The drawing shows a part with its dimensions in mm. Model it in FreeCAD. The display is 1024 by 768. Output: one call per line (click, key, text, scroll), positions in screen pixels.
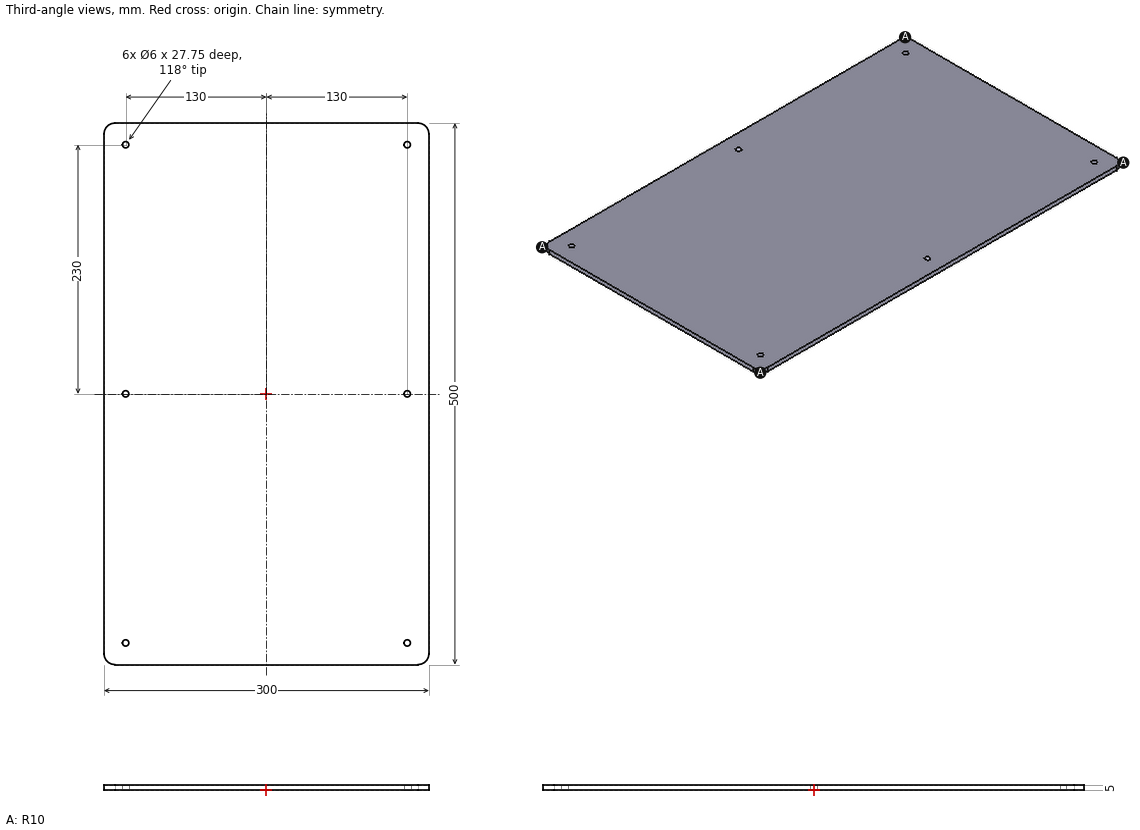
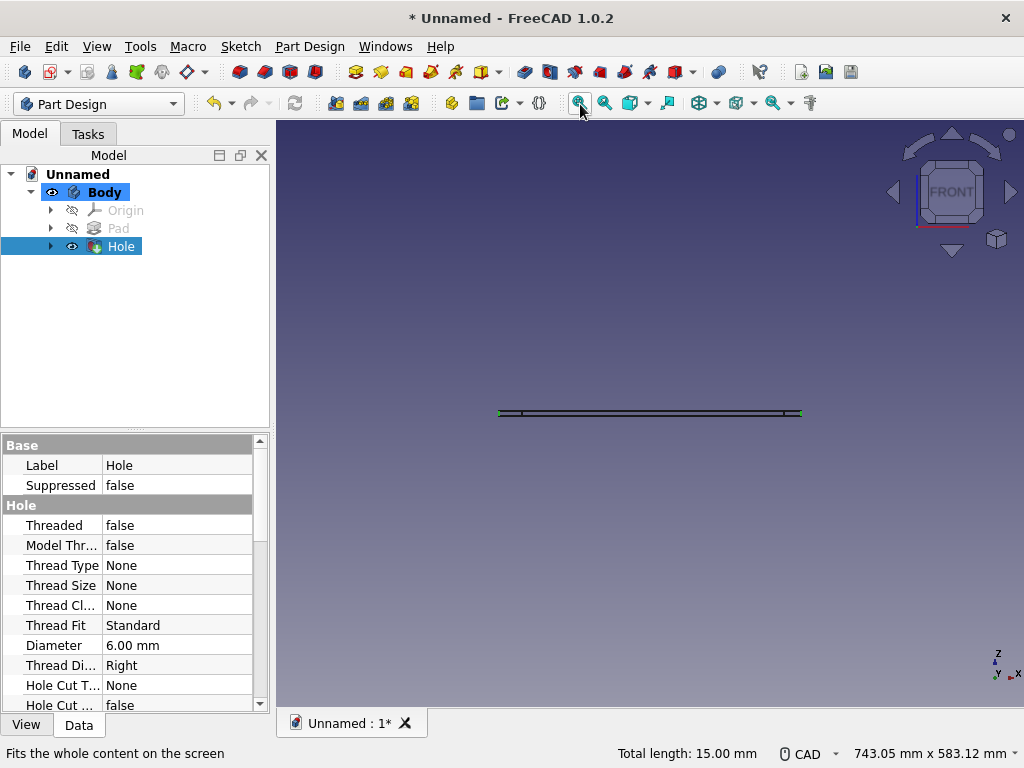
click(580, 104)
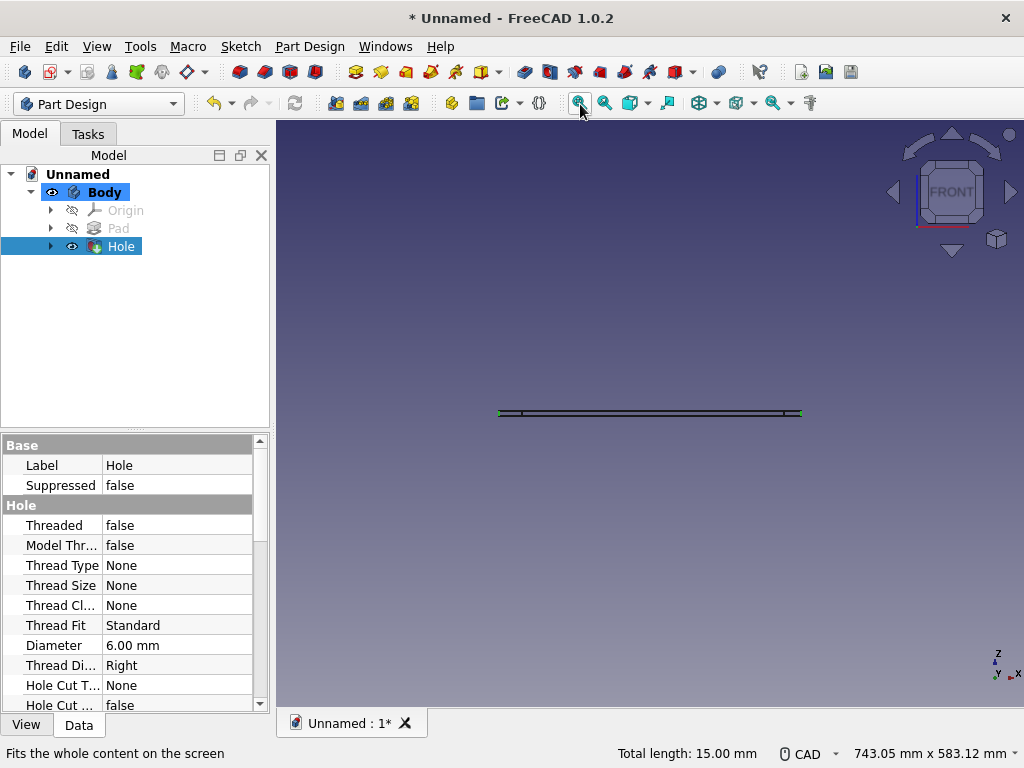
scroll(801, 413, up, 11)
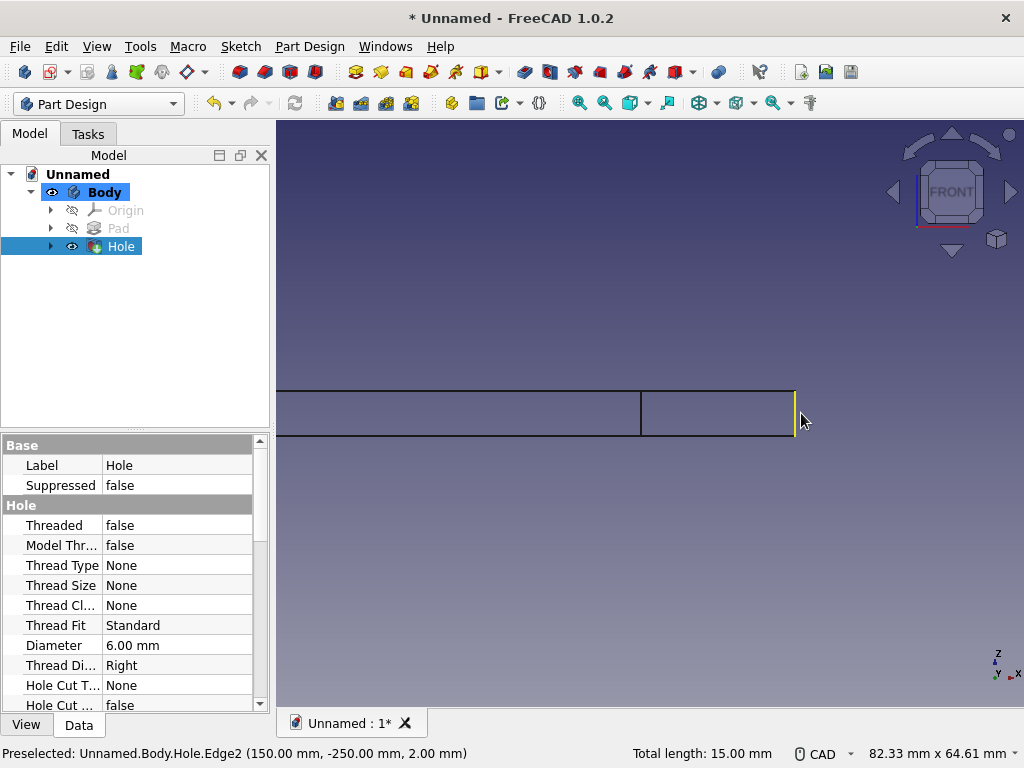
click(580, 104)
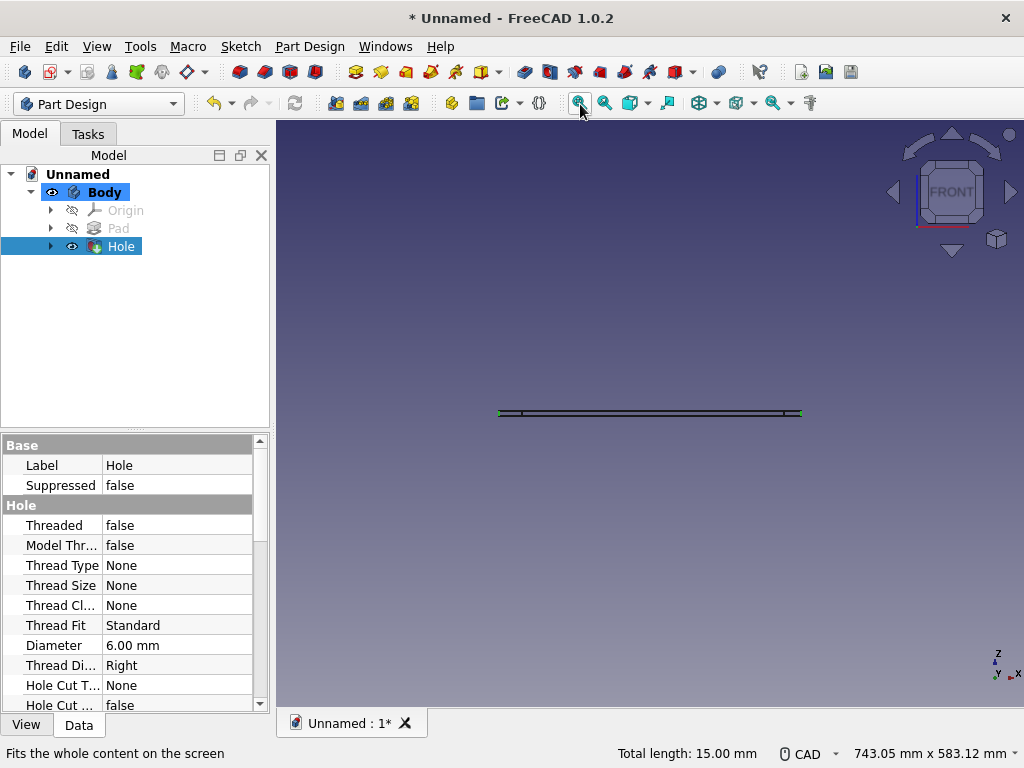
key(3)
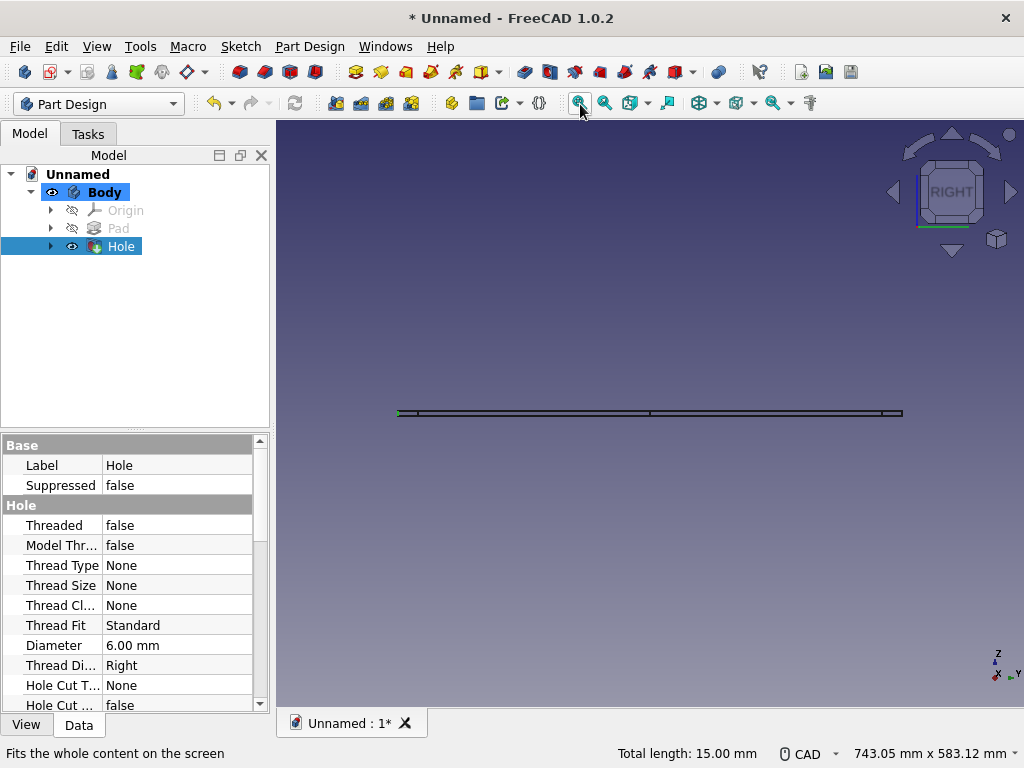
key(5)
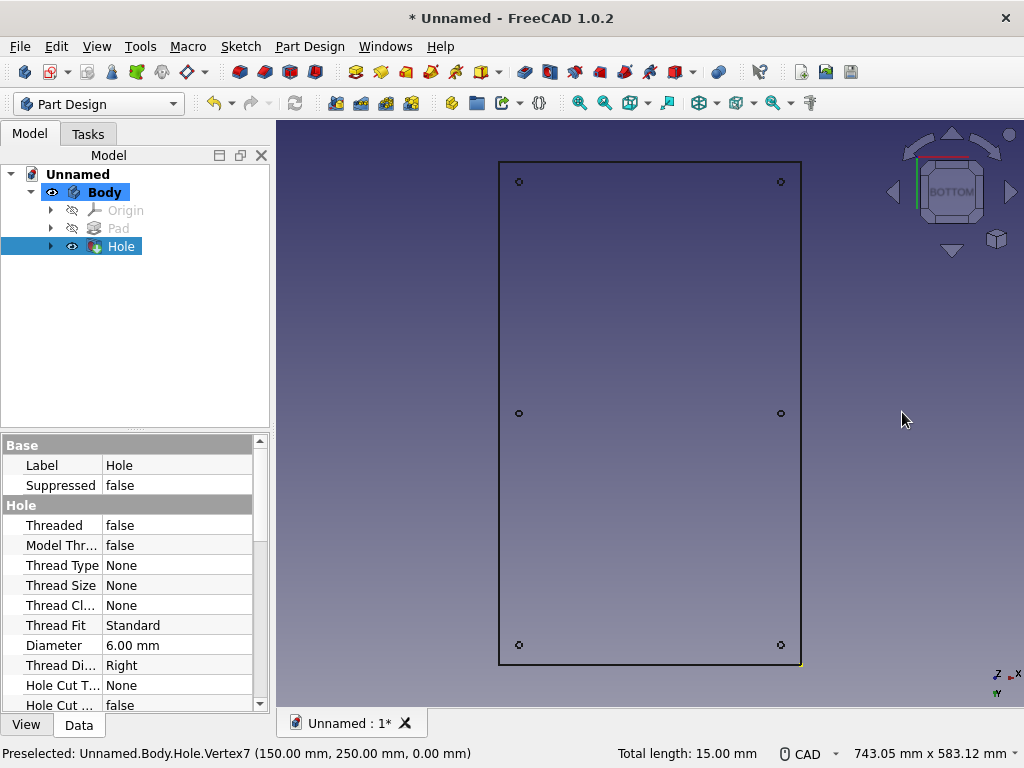
scroll(801, 664, up, 11)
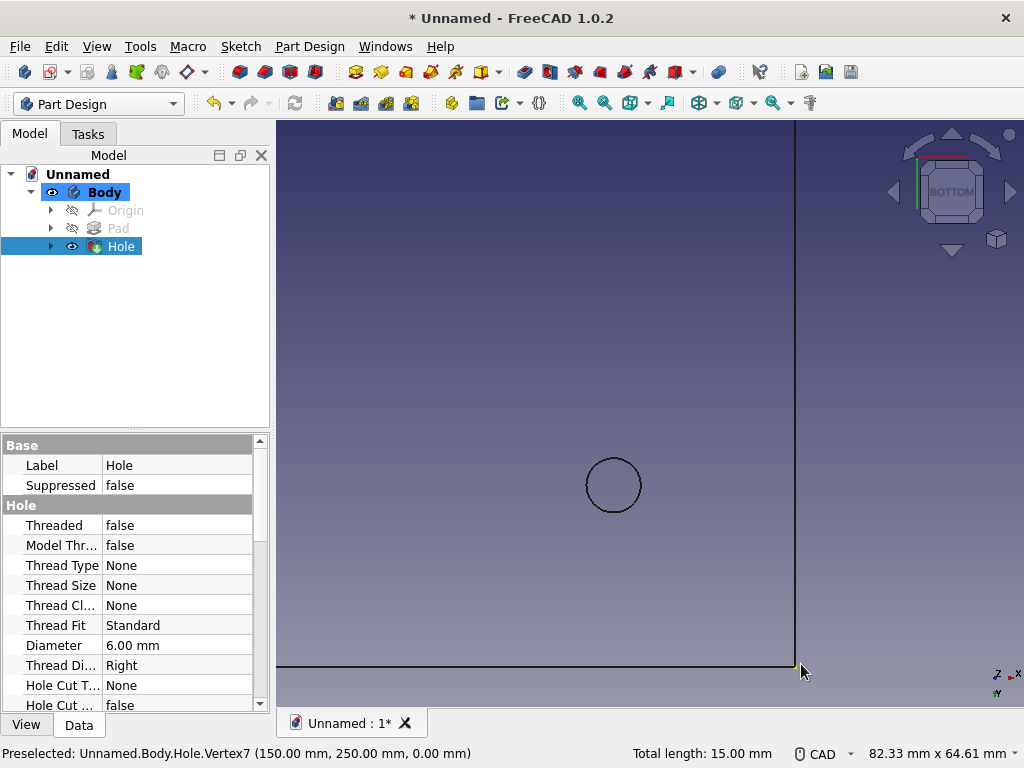
click(580, 104)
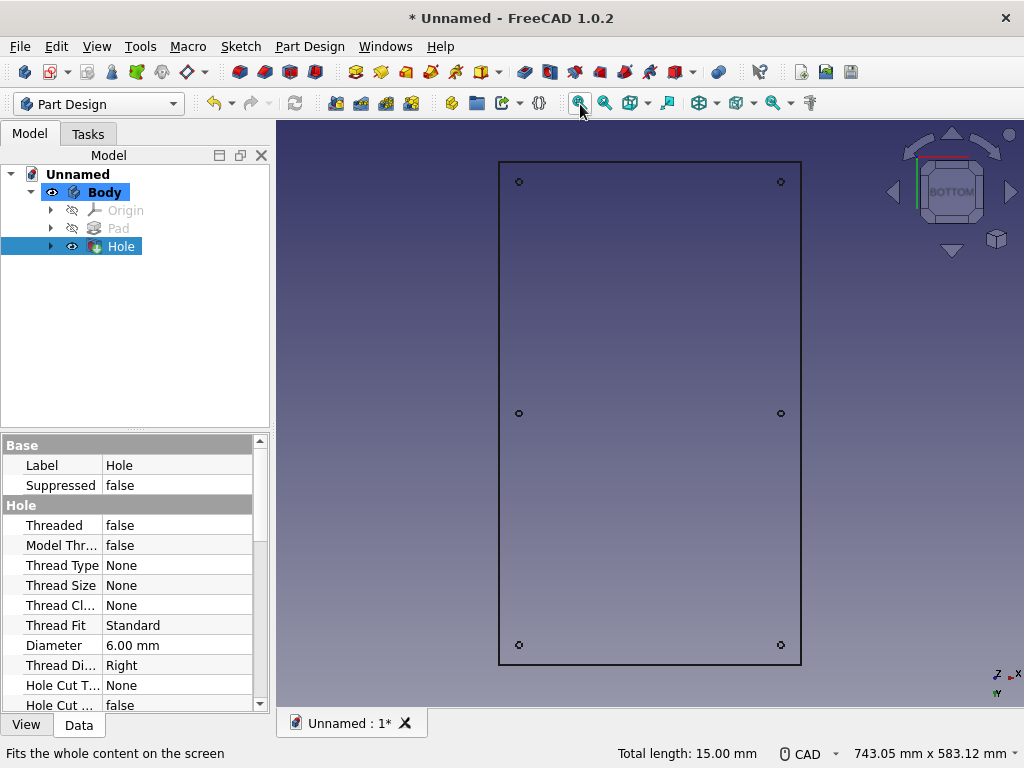
key(4)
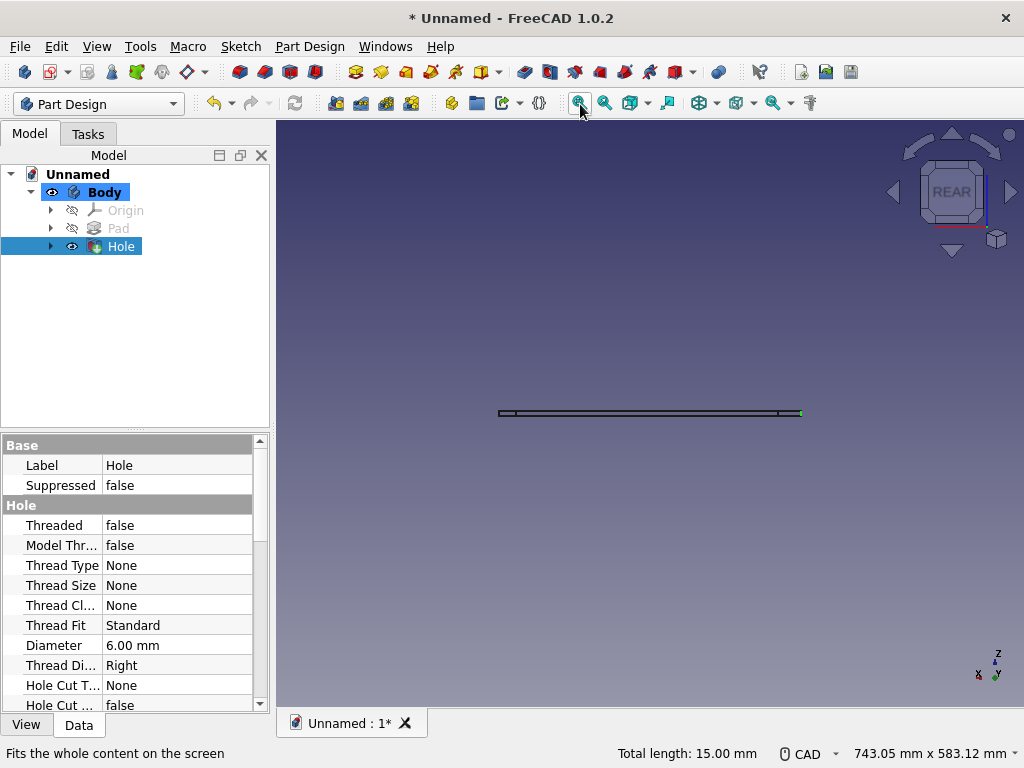
click(580, 104)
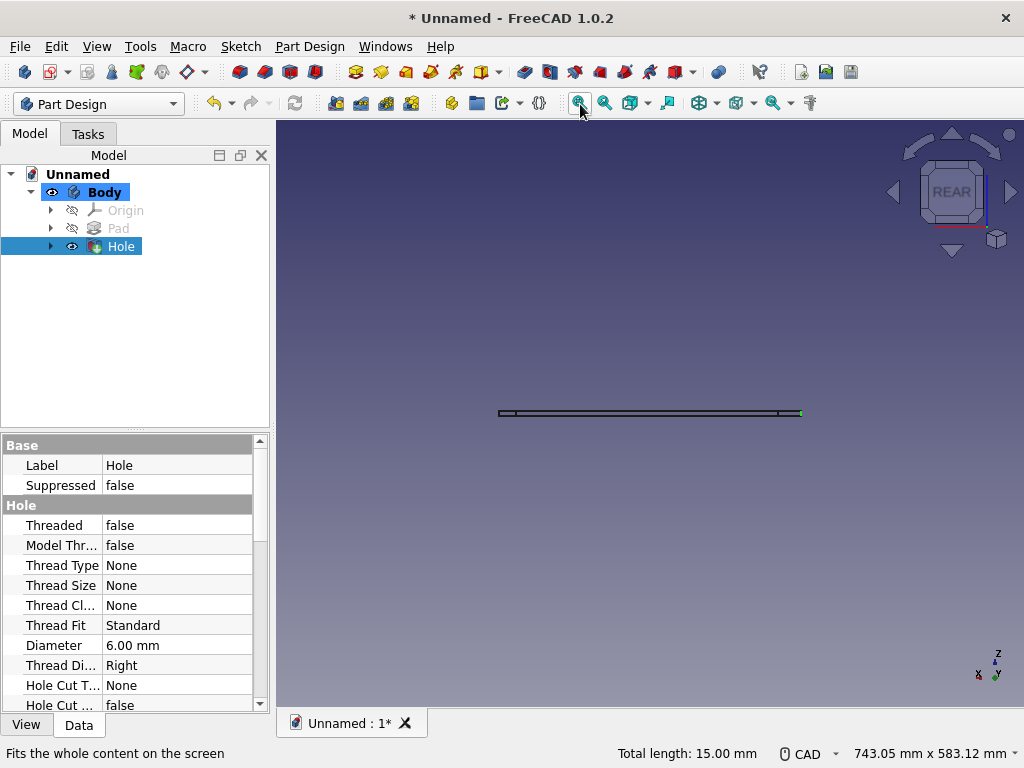
scroll(499, 413, up, 11)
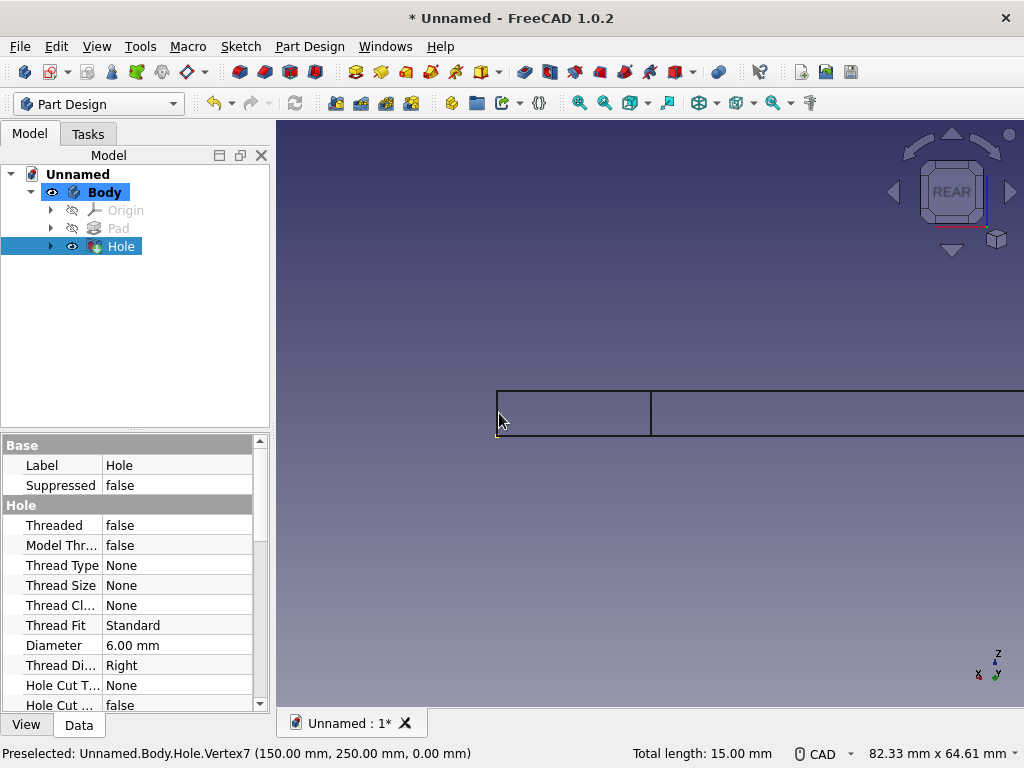
click(497, 413, ctrl)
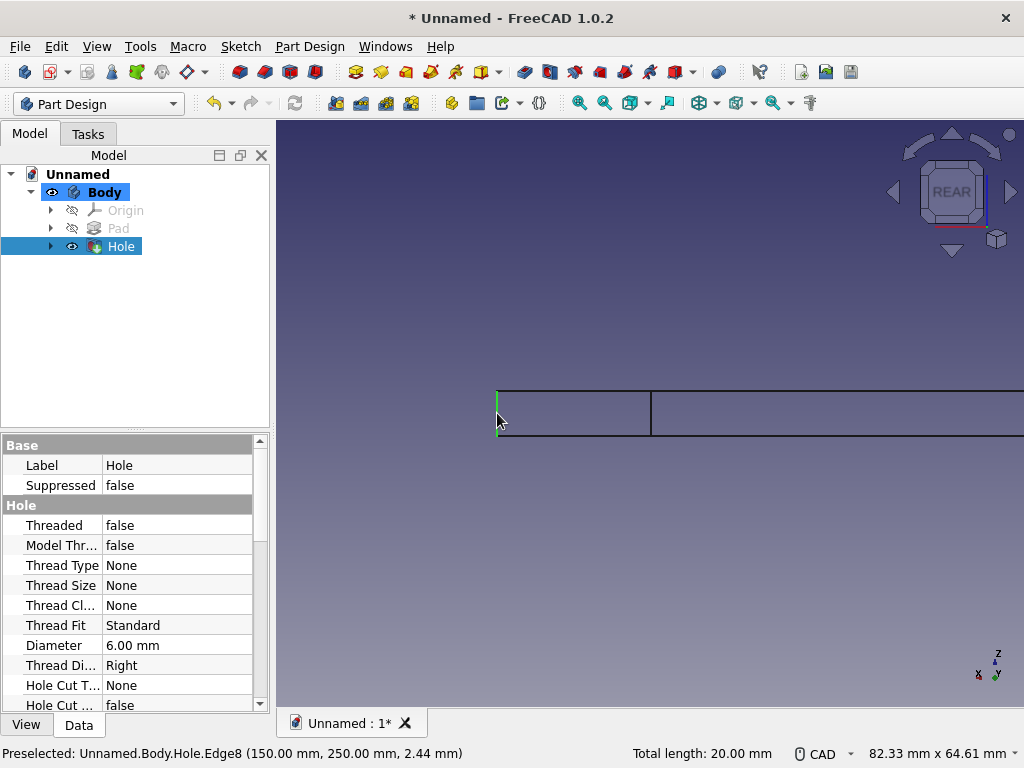
key(v)
key(1)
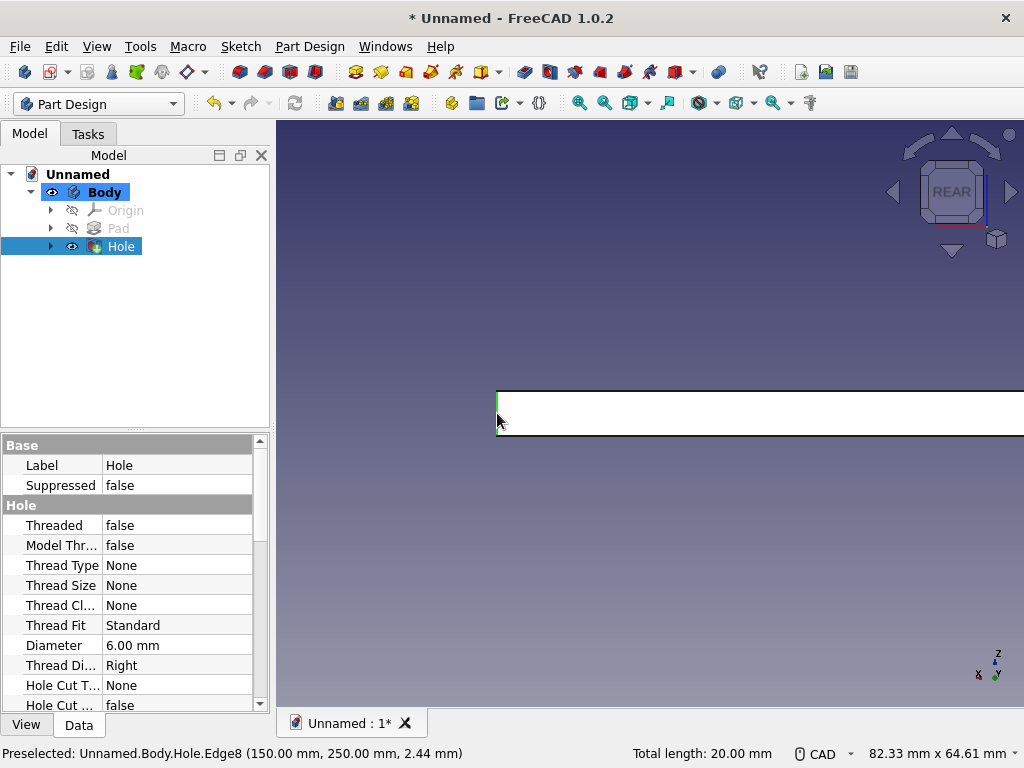
click(240, 72)